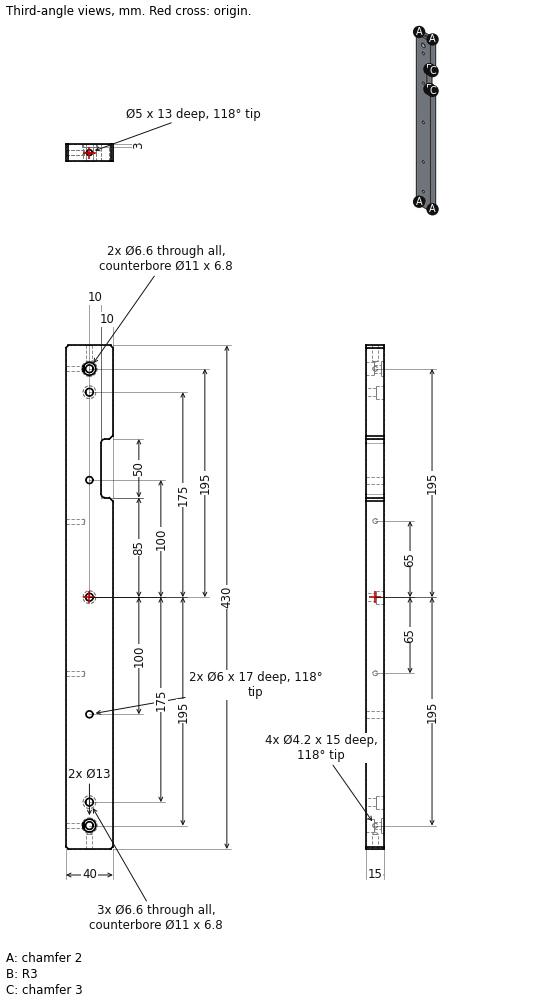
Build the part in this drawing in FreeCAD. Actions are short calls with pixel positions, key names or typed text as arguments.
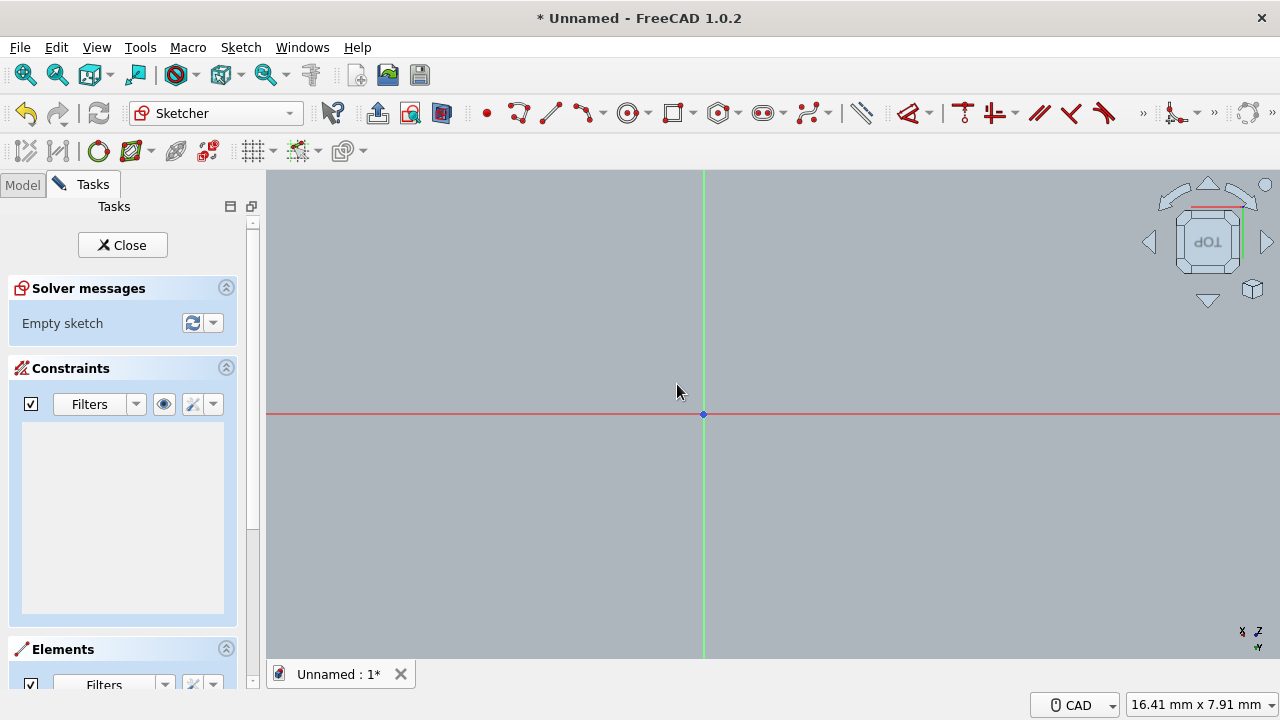
click(628, 114)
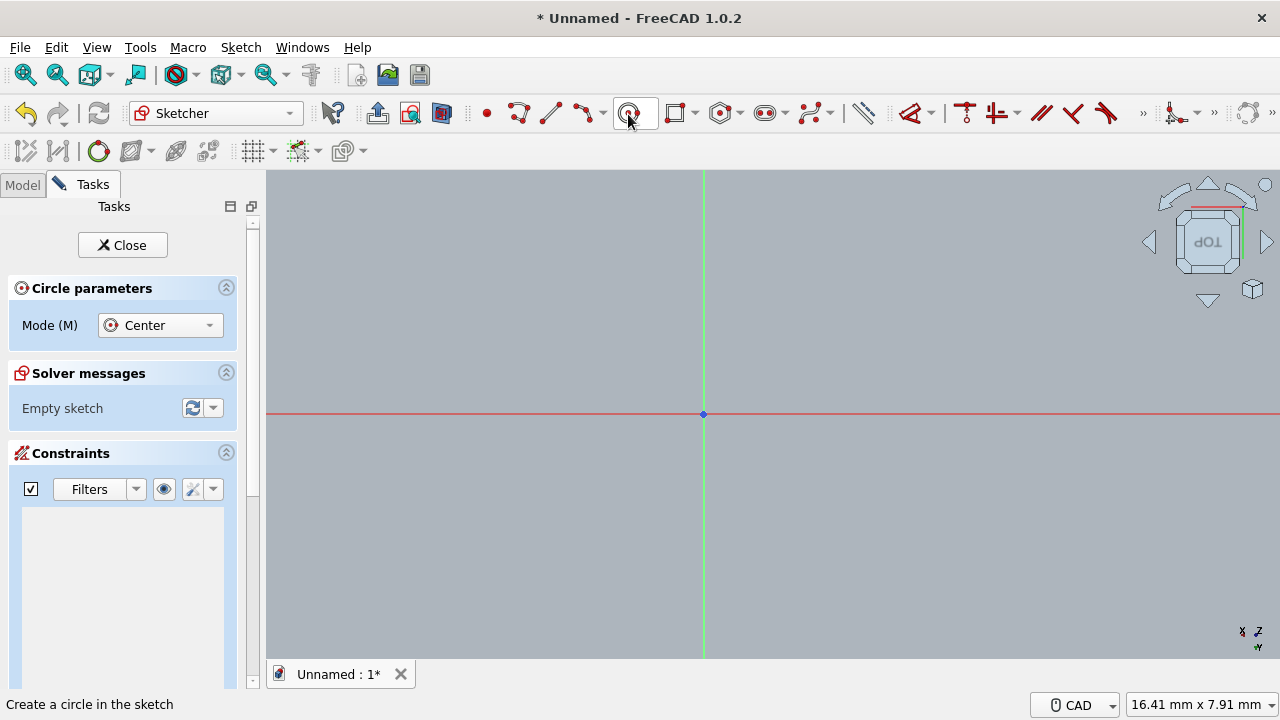
click(704, 414)
move(813, 305)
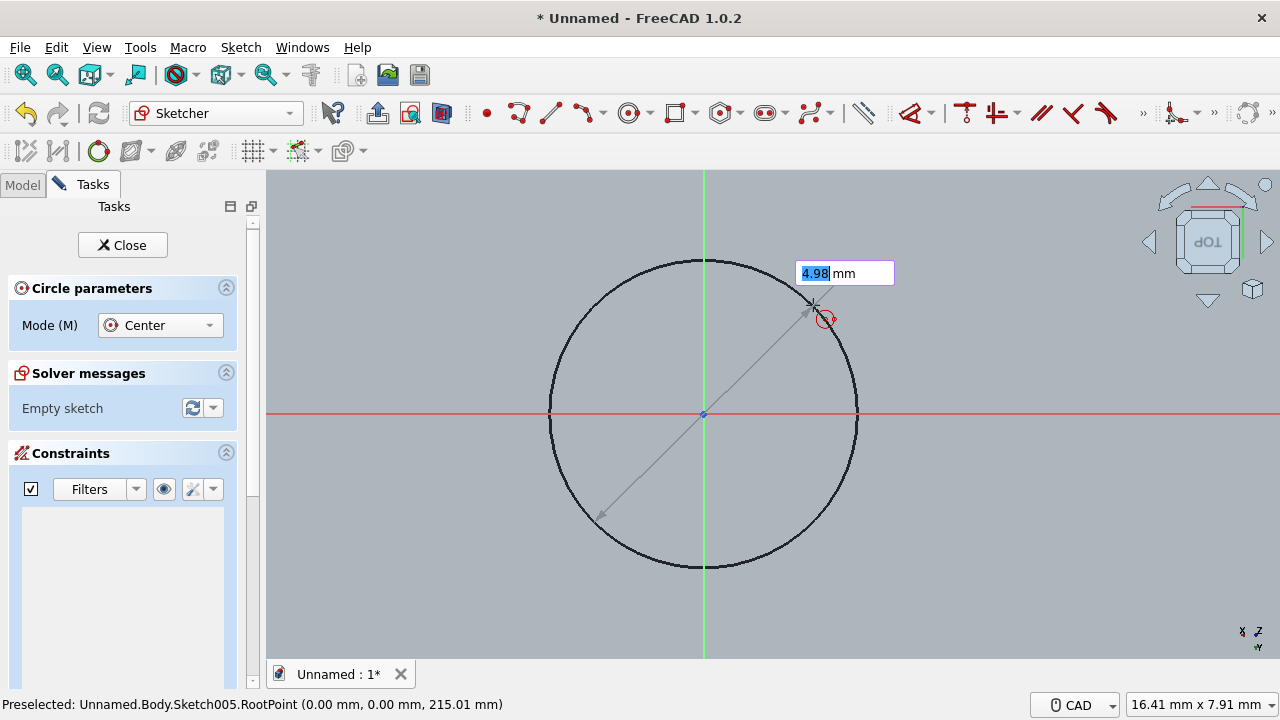
text(5)
key(Return)
key(Escape)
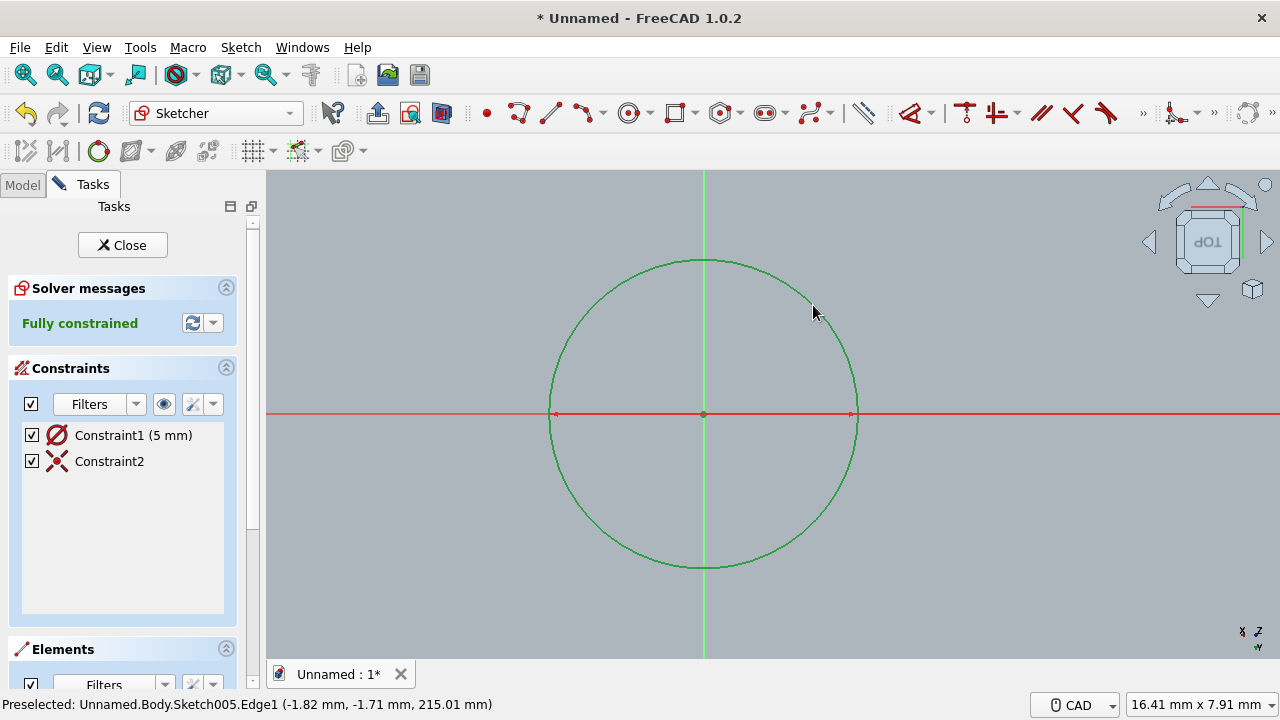
click(123, 245)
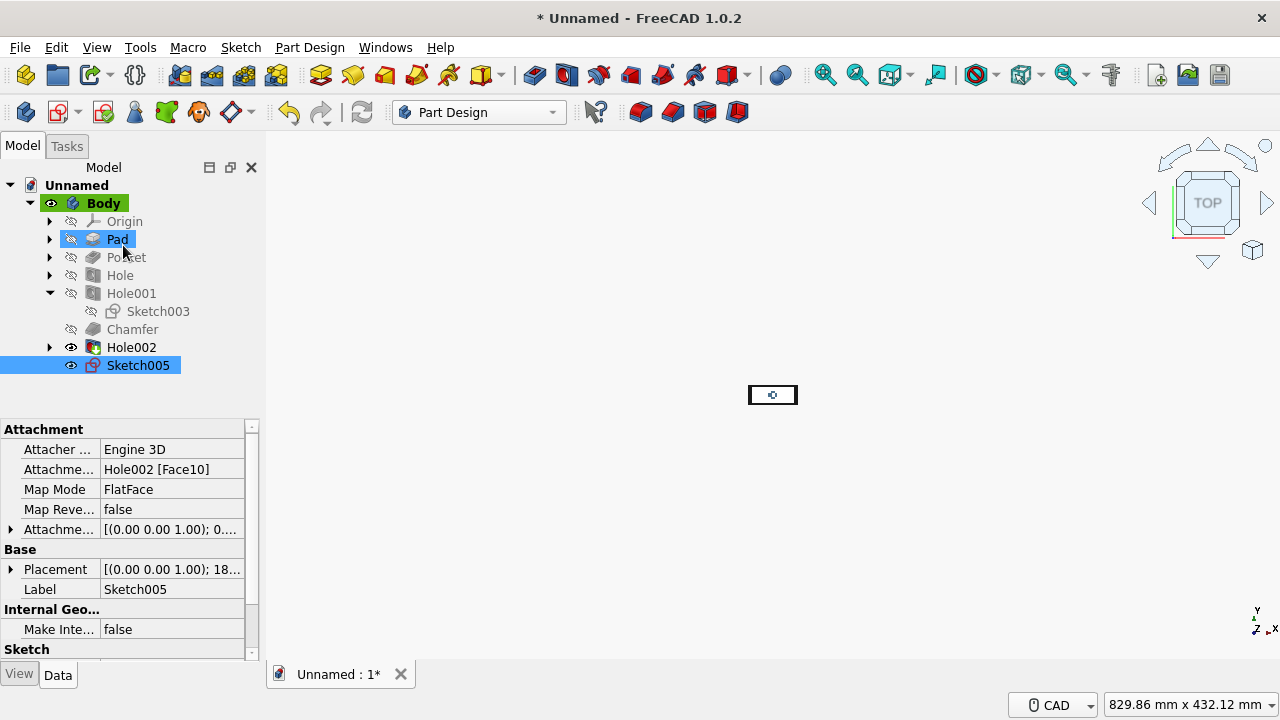
click(568, 76)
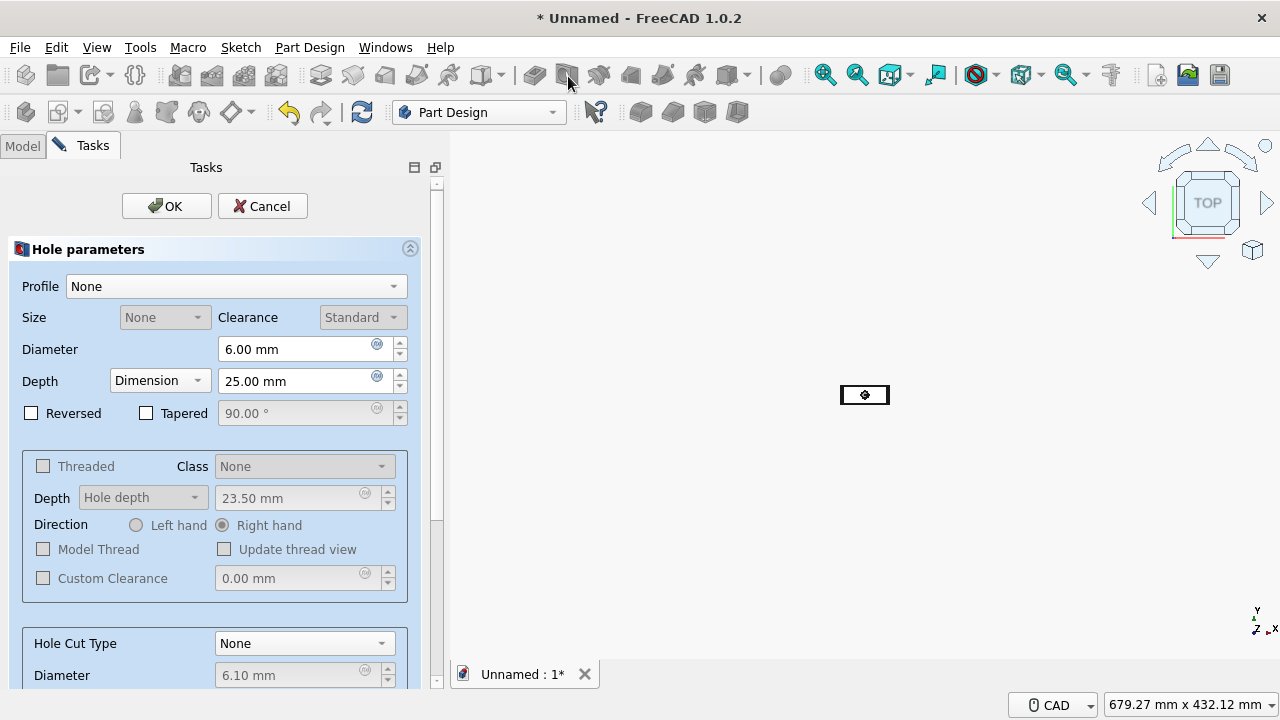
triple_click(305, 349)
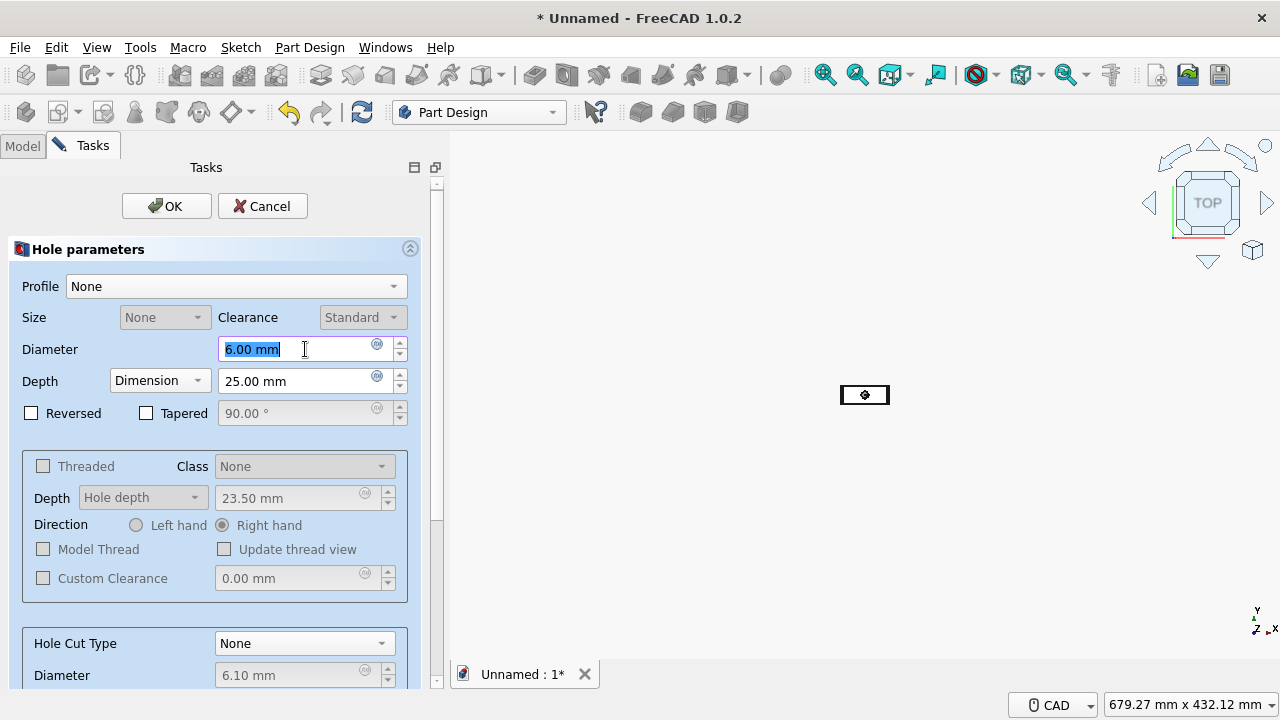
text(5)
key(Tab)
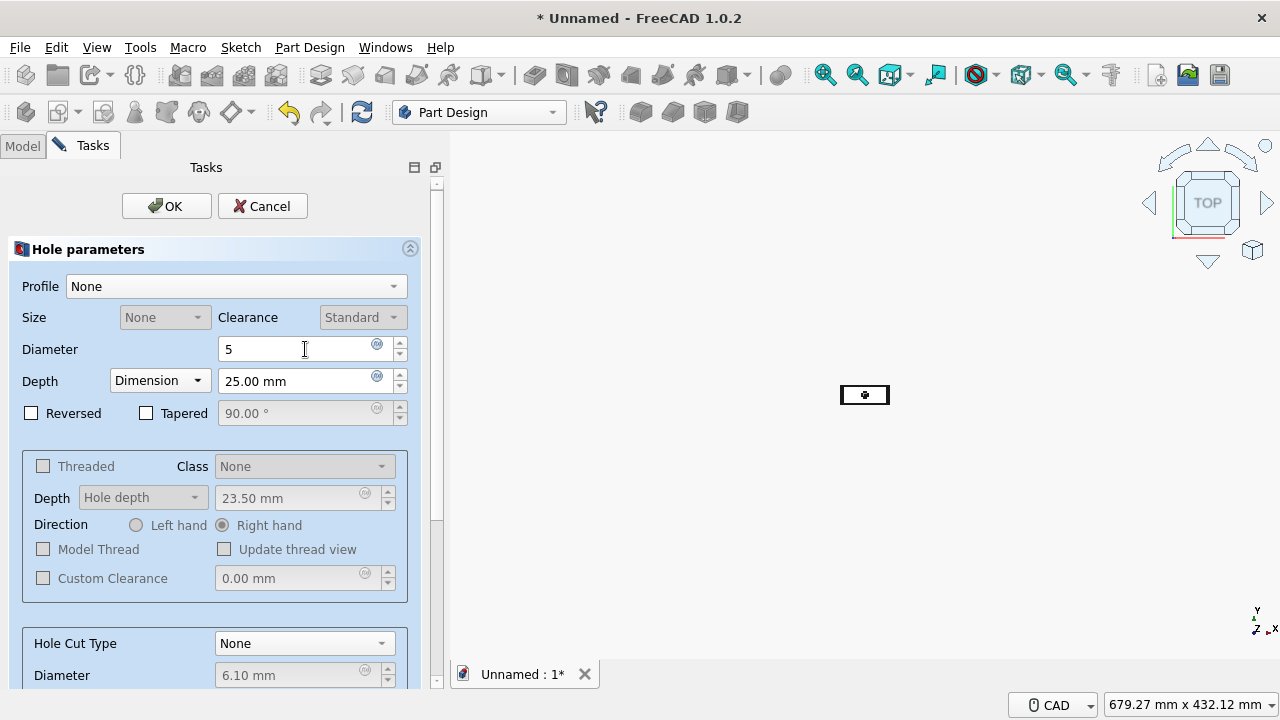
triple_click(305, 381)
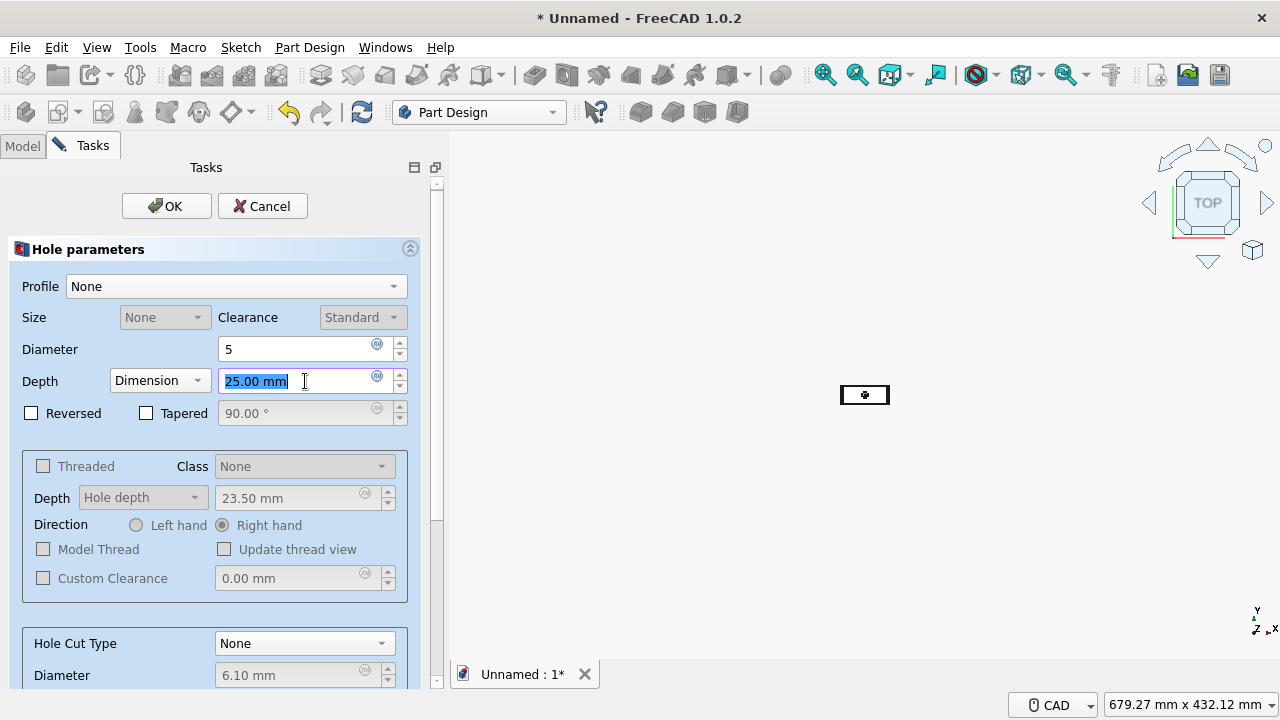
text(13)
key(Tab)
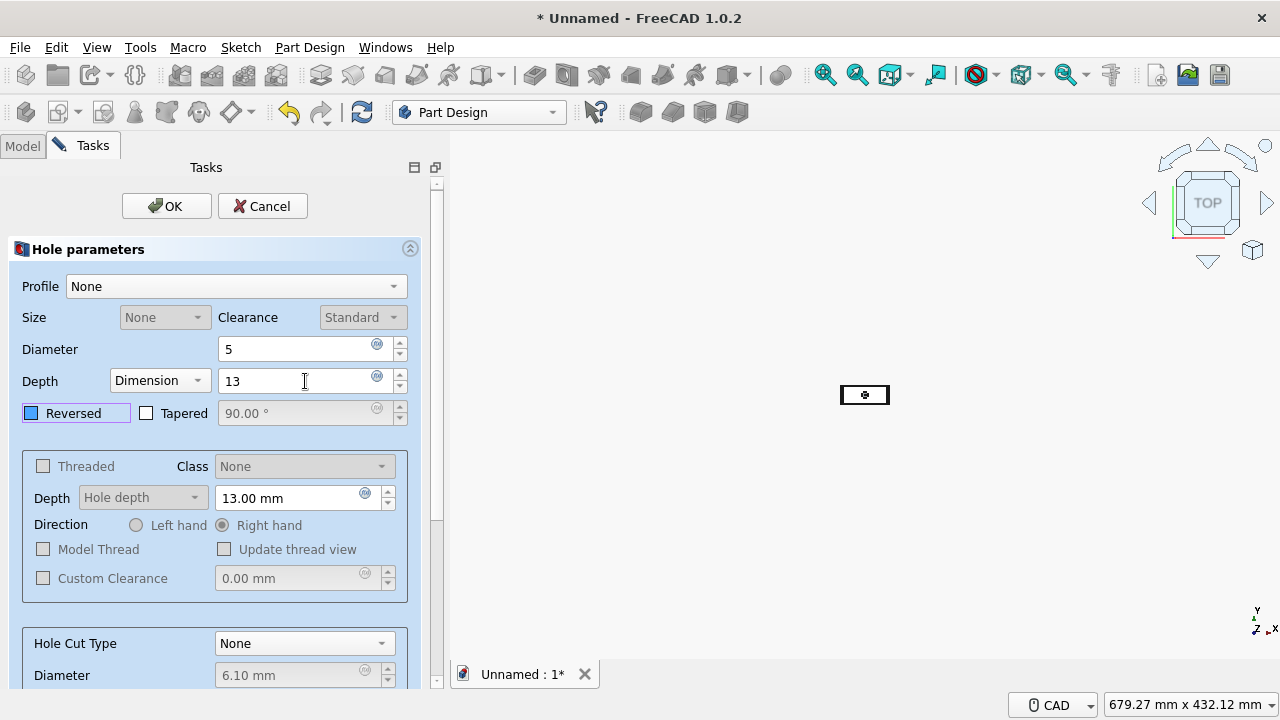
click(167, 206)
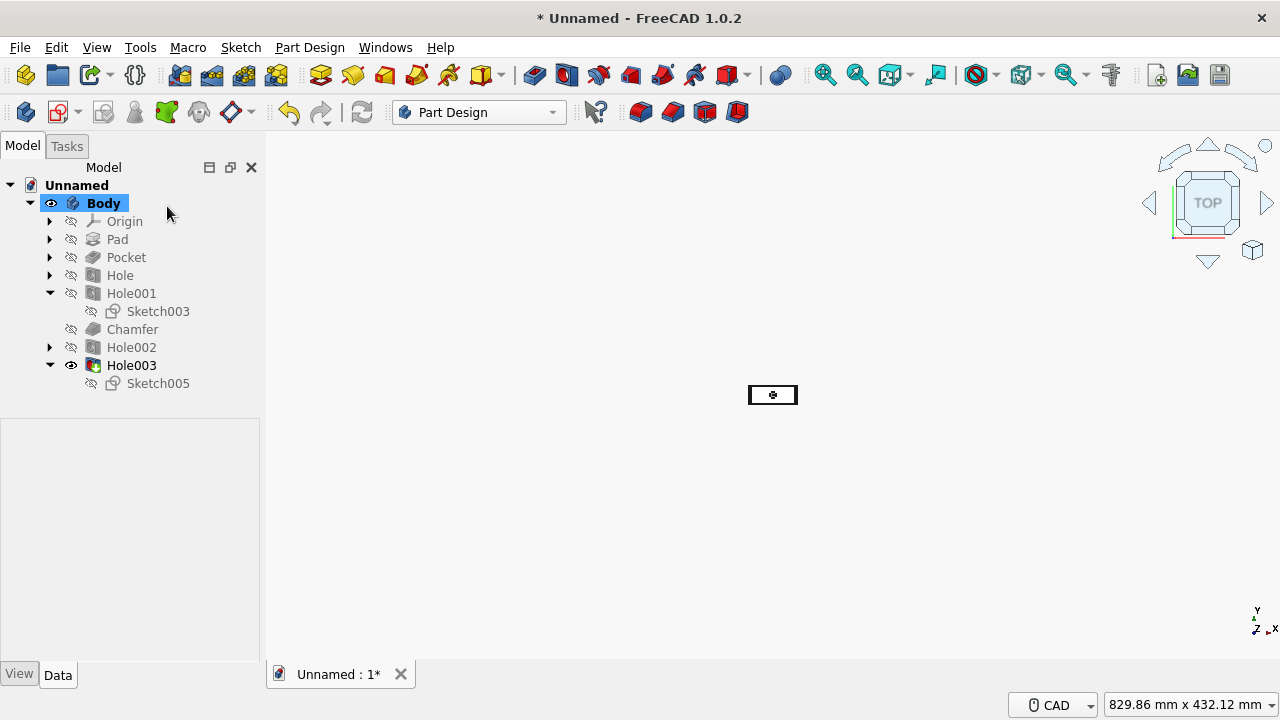
click(826, 76)